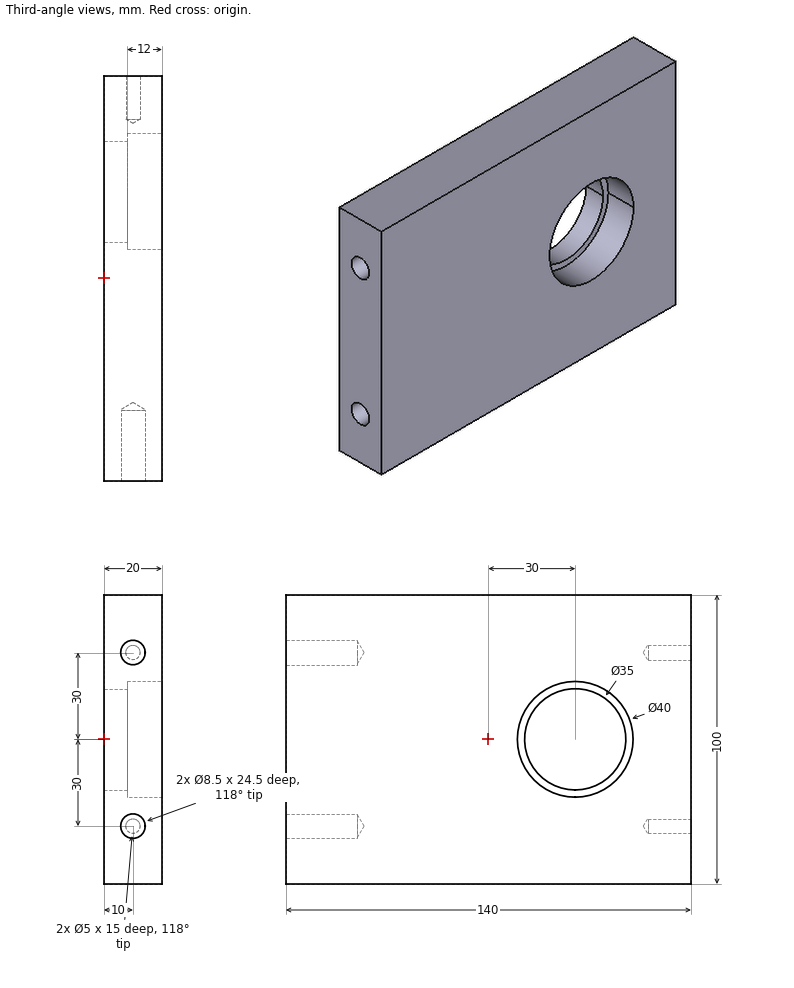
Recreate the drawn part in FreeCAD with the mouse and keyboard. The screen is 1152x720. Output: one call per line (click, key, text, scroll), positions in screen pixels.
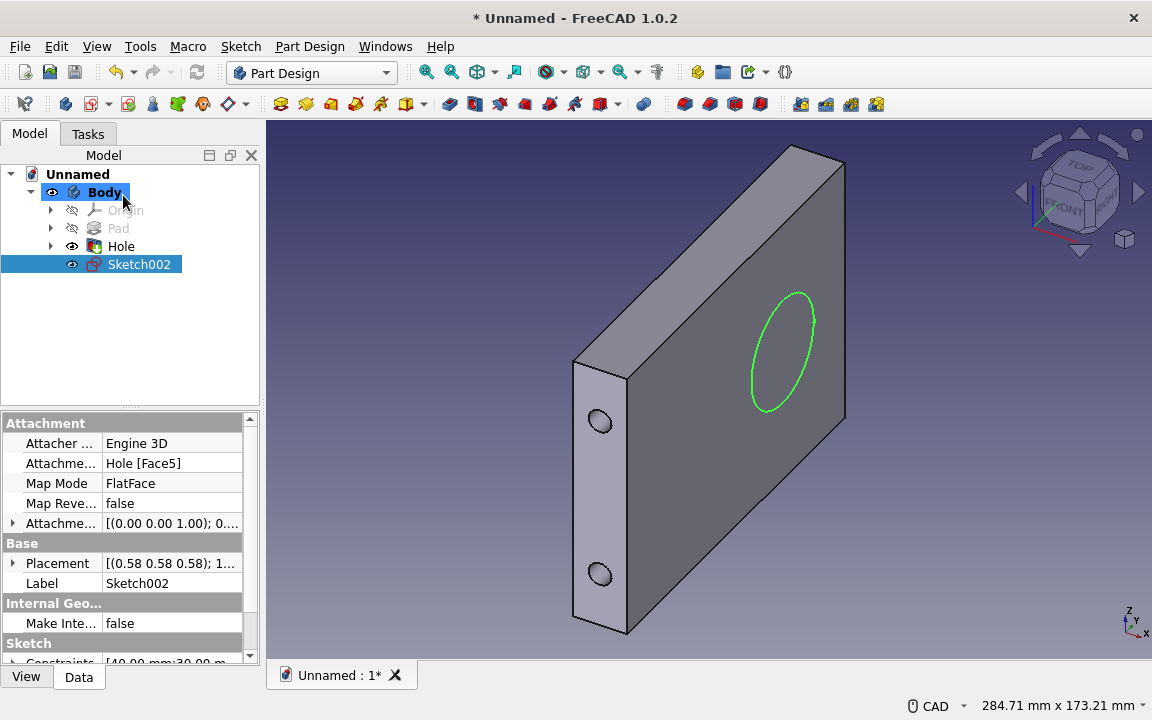
click(450, 104)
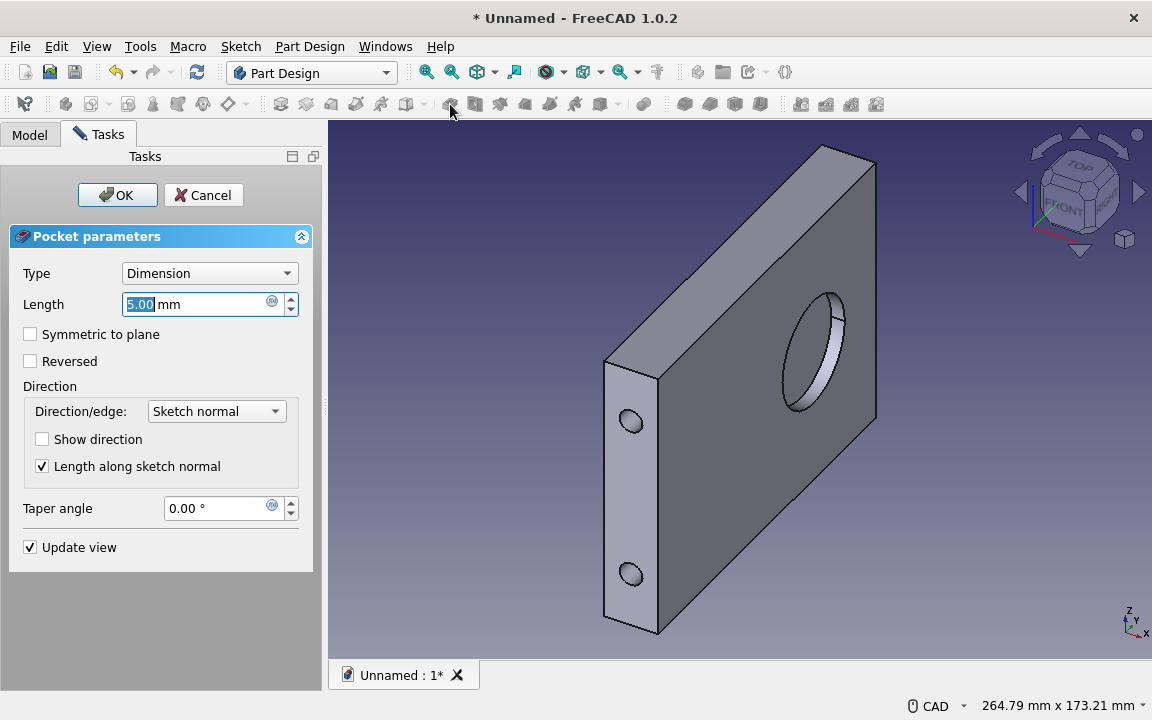
text(12)
key(Tab)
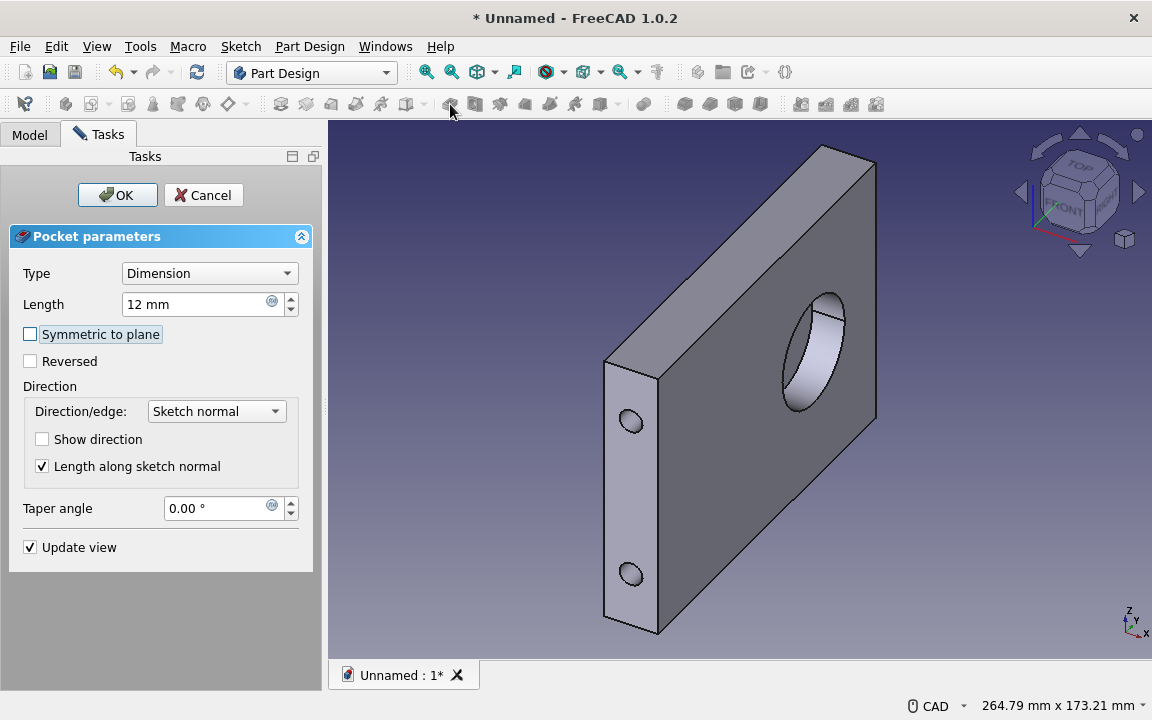
click(118, 195)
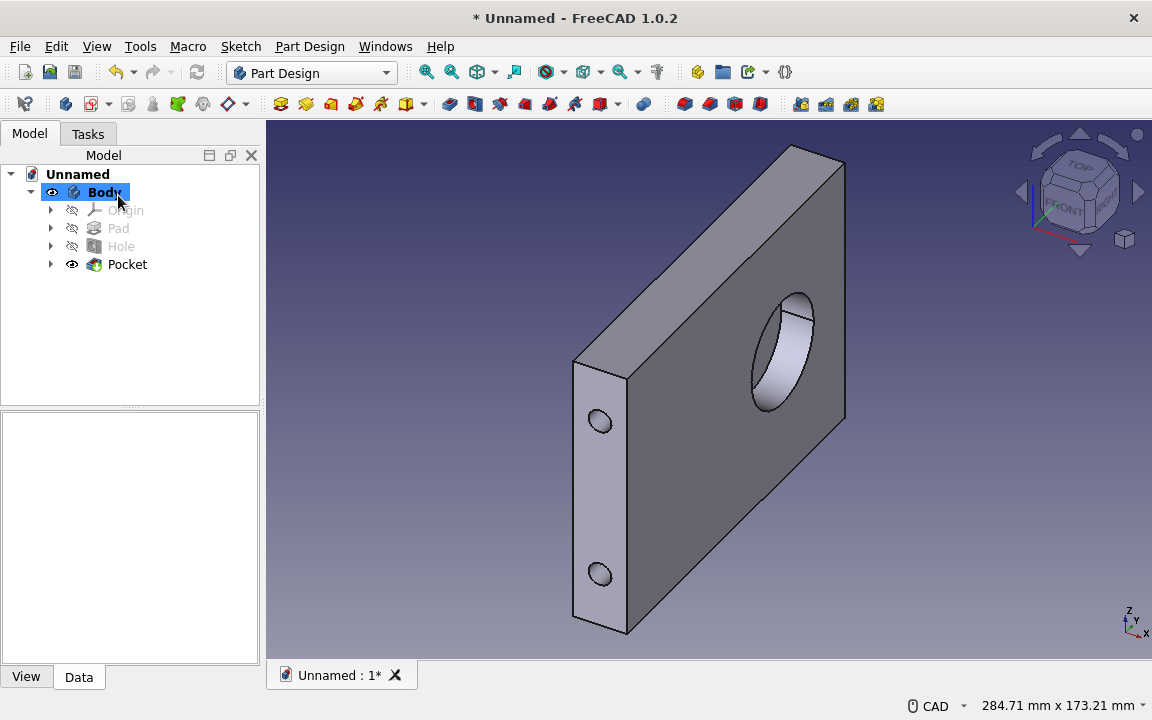
key(0)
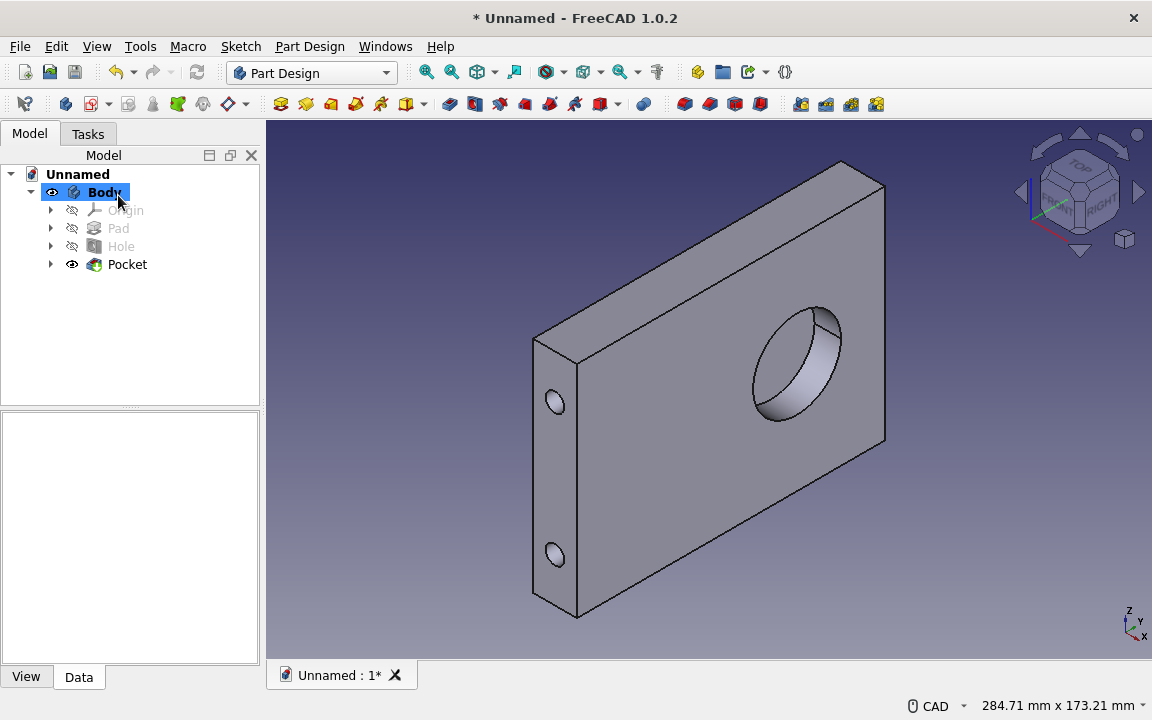
click(783, 341)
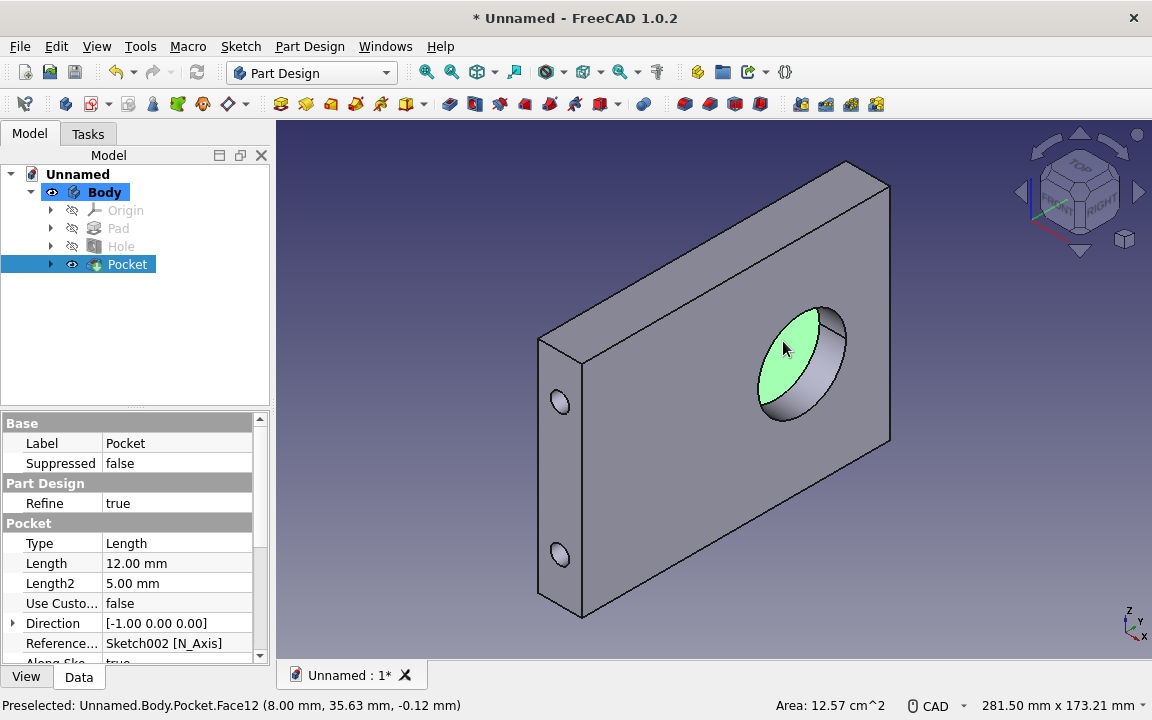
click(90, 104)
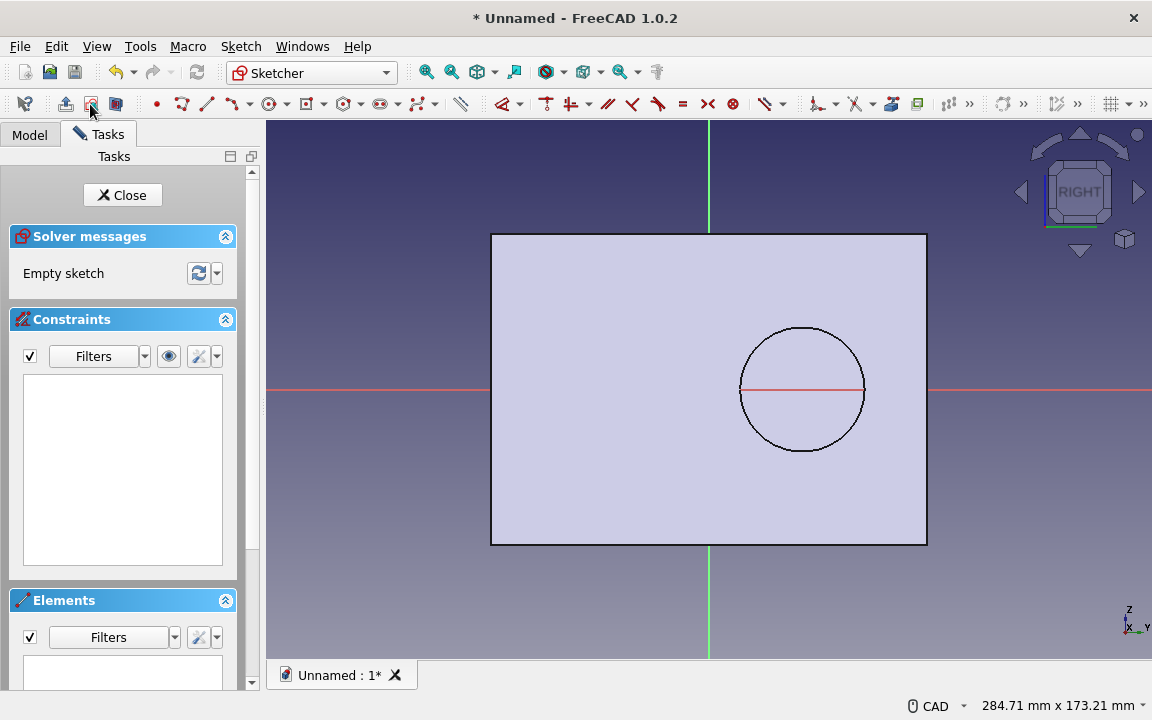
scroll(844, 389, up, 6)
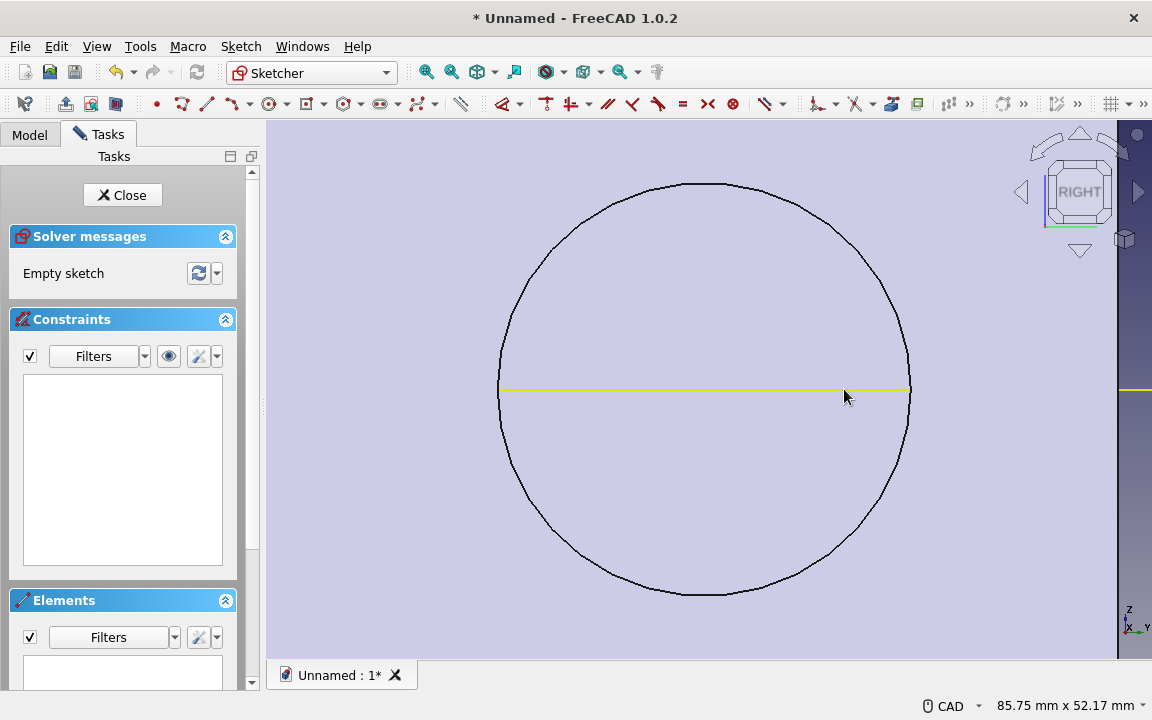
click(268, 104)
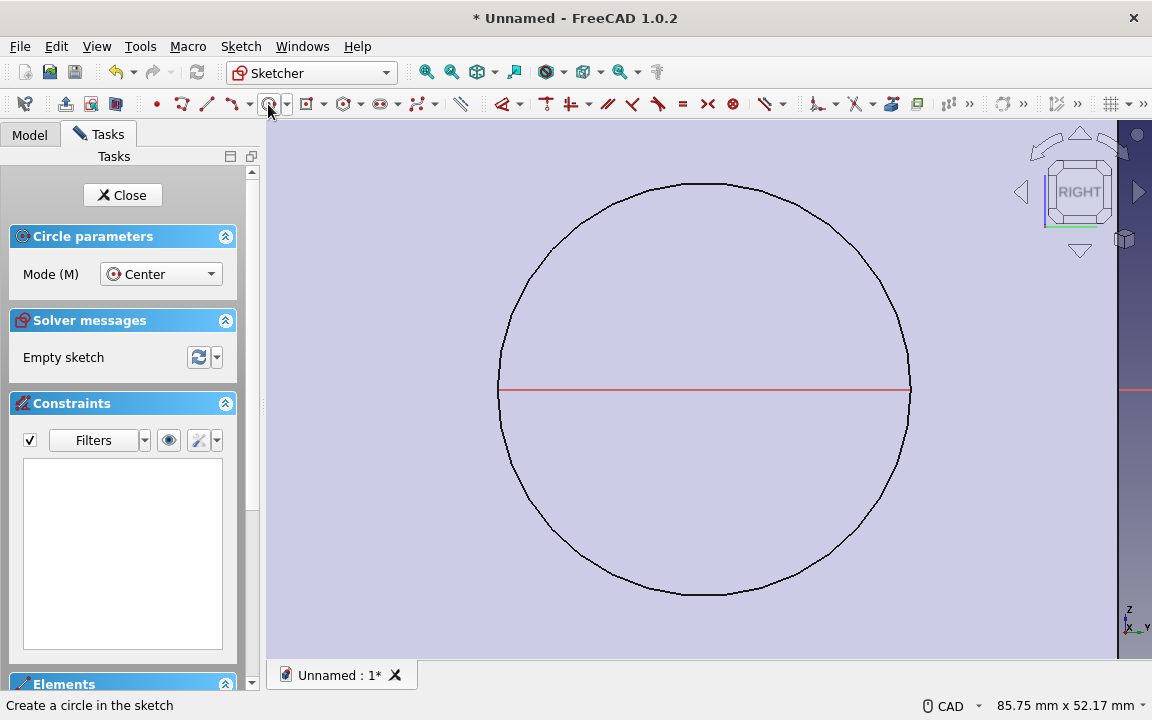
click(704, 389)
move(832, 262)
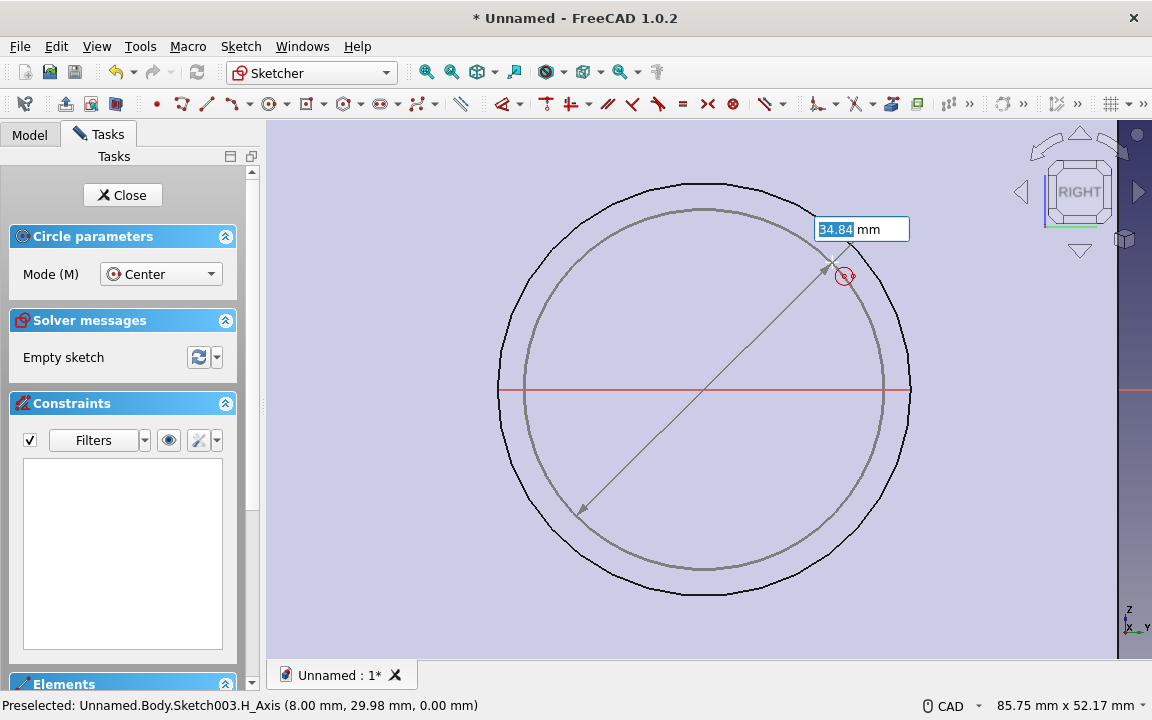
text(35)
key(Return)
key(Escape)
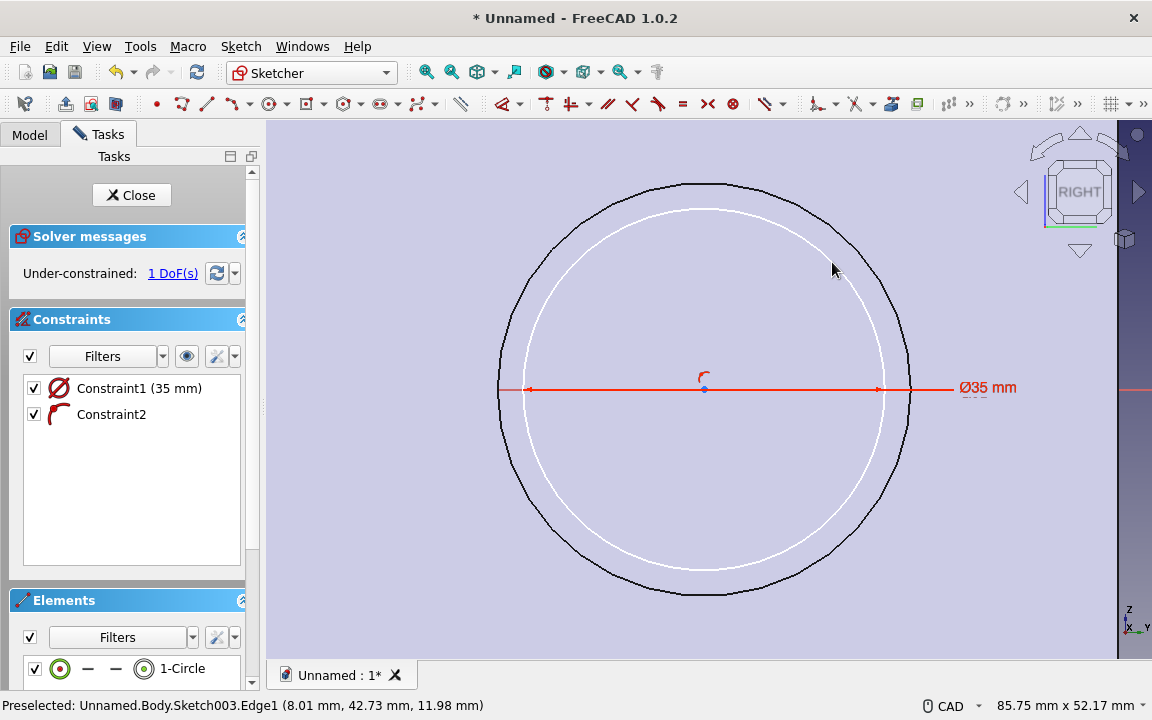
key(d)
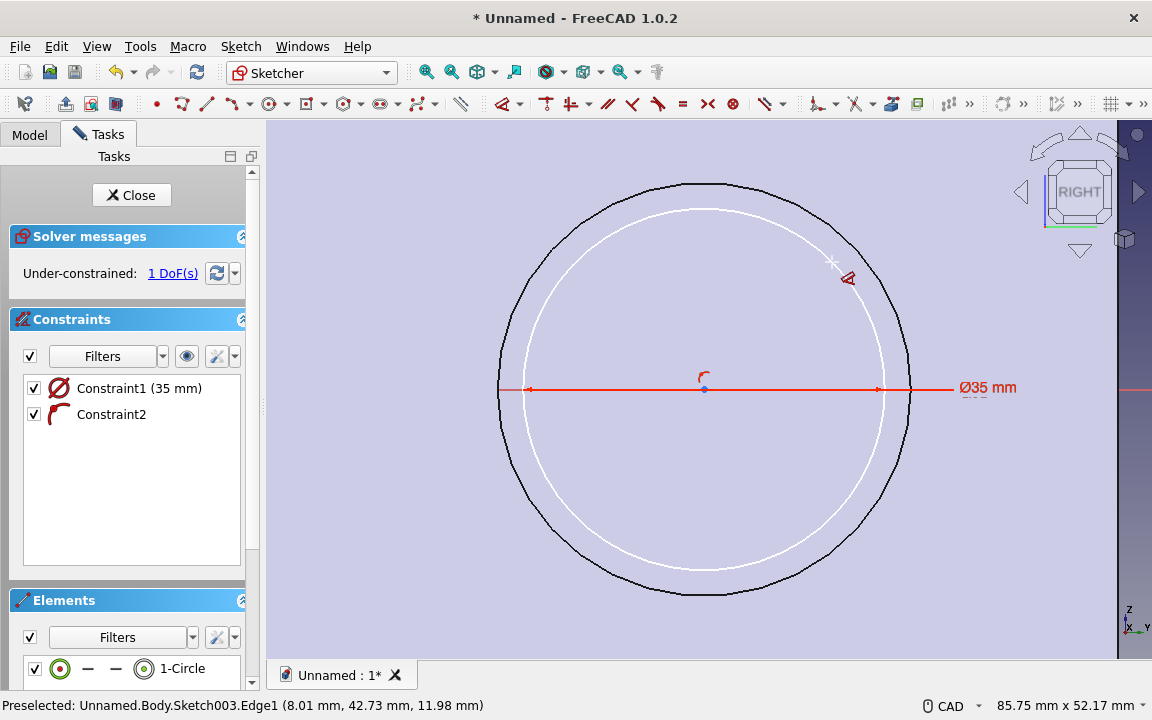
click(704, 389)
click(549, 423)